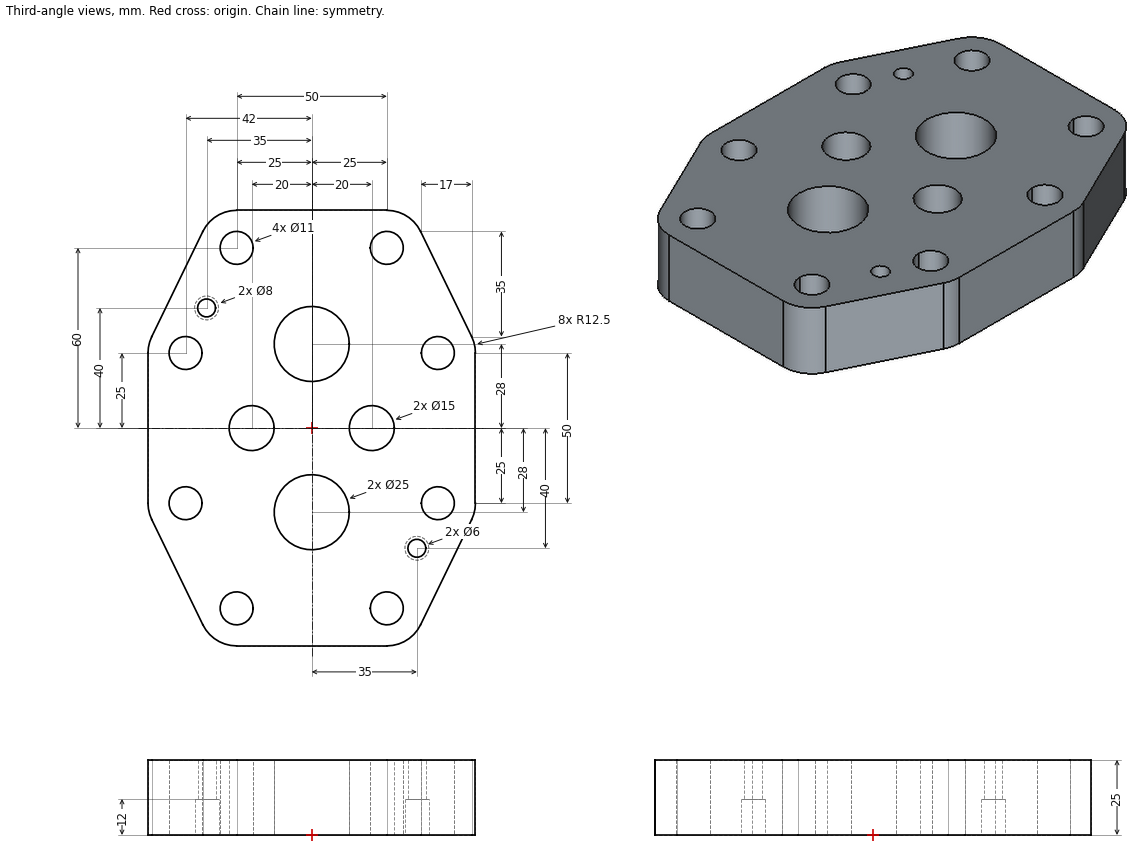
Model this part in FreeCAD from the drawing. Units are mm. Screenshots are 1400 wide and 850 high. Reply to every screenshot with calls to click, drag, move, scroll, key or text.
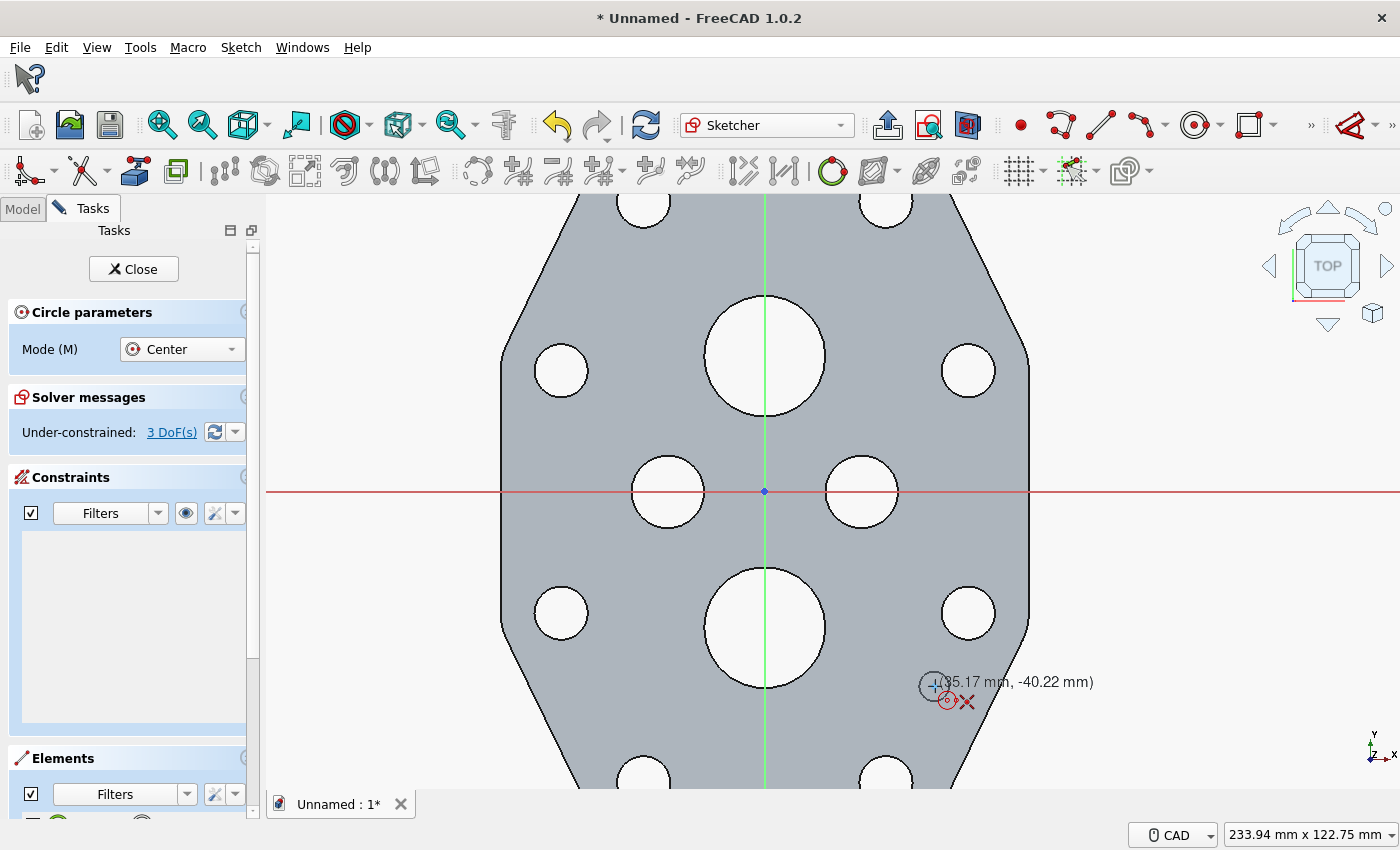
scroll(595, 298, up, 3)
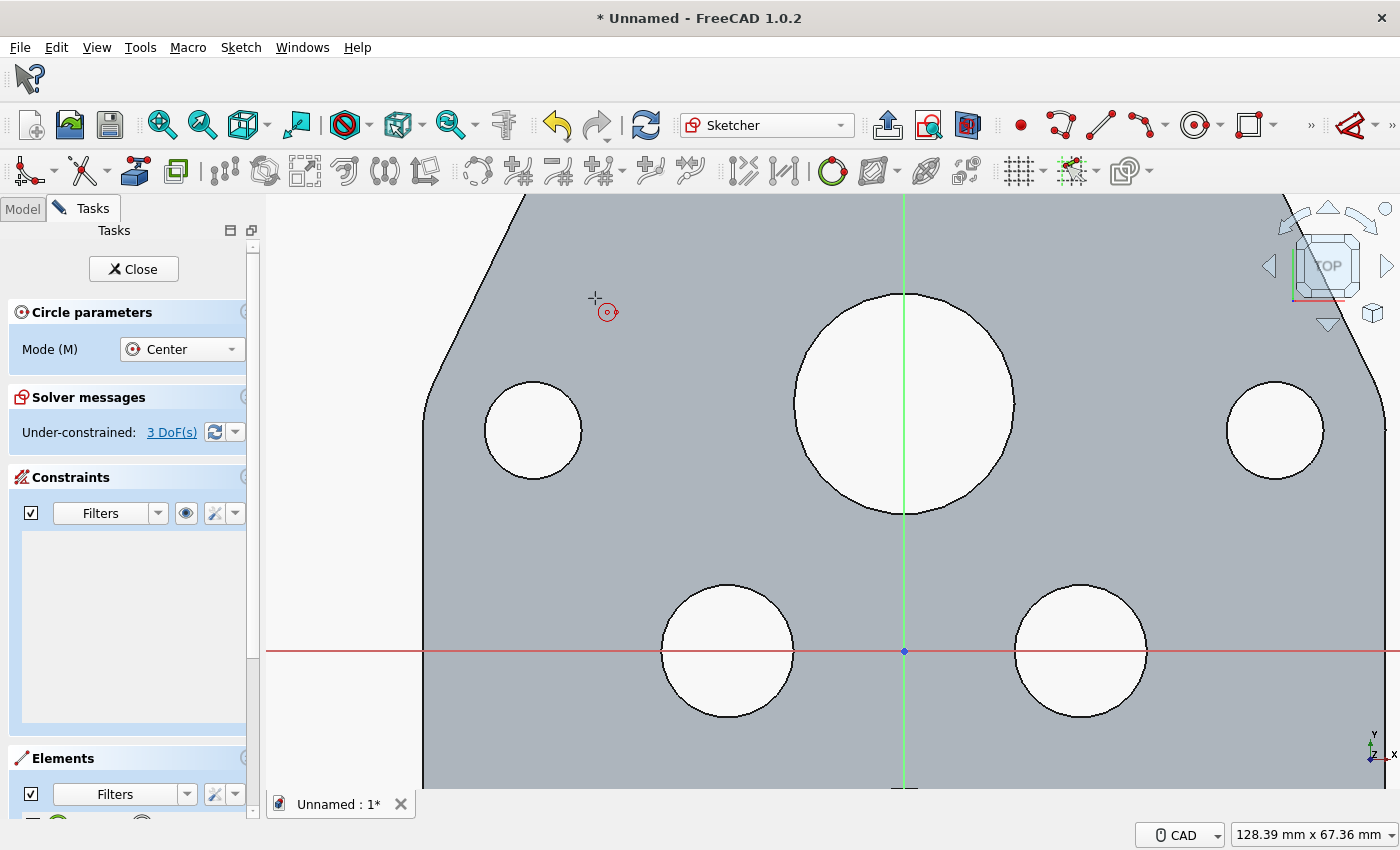
click(595, 298)
click(614, 279)
key(Escape)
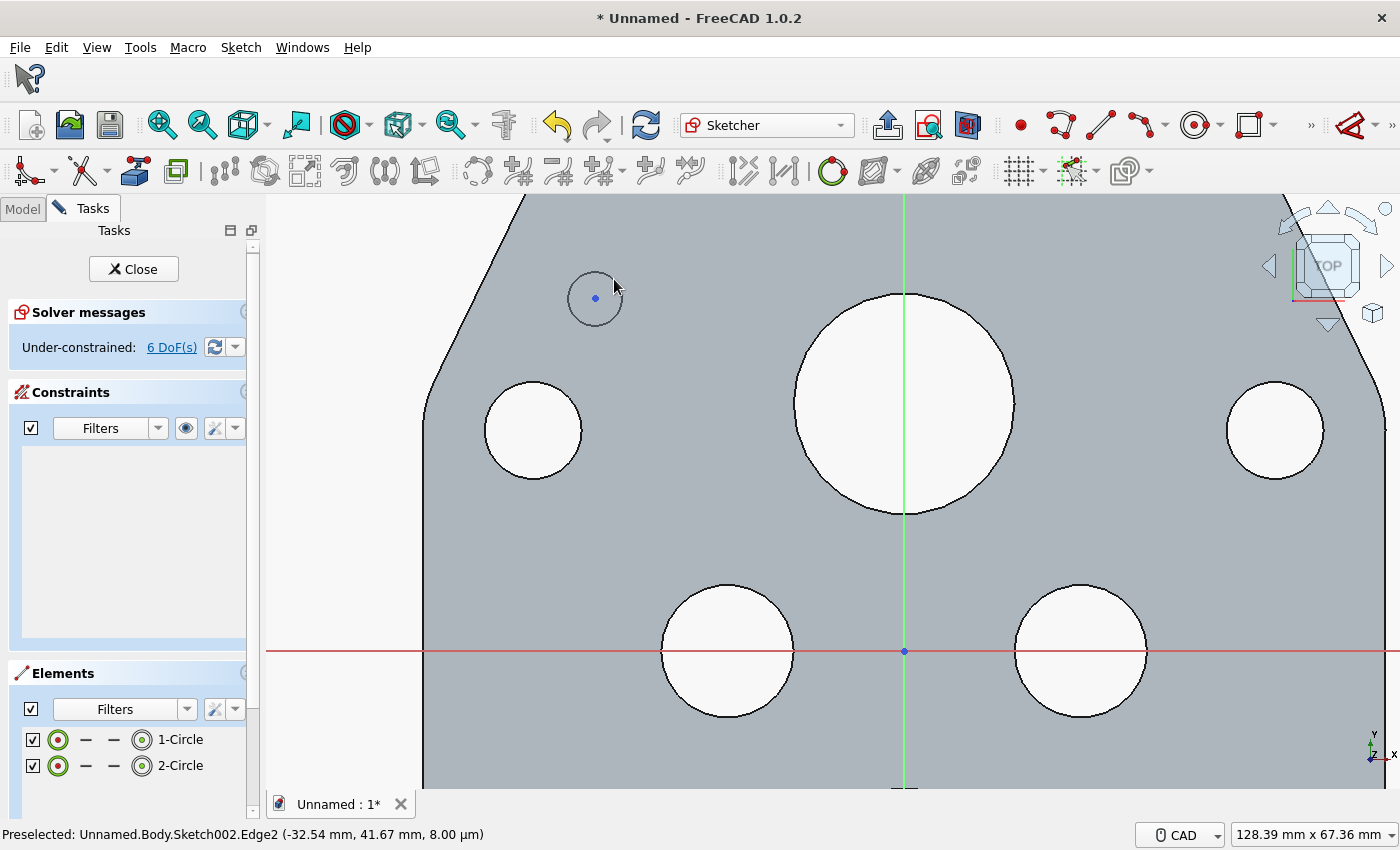
scroll(595, 297, down, 3)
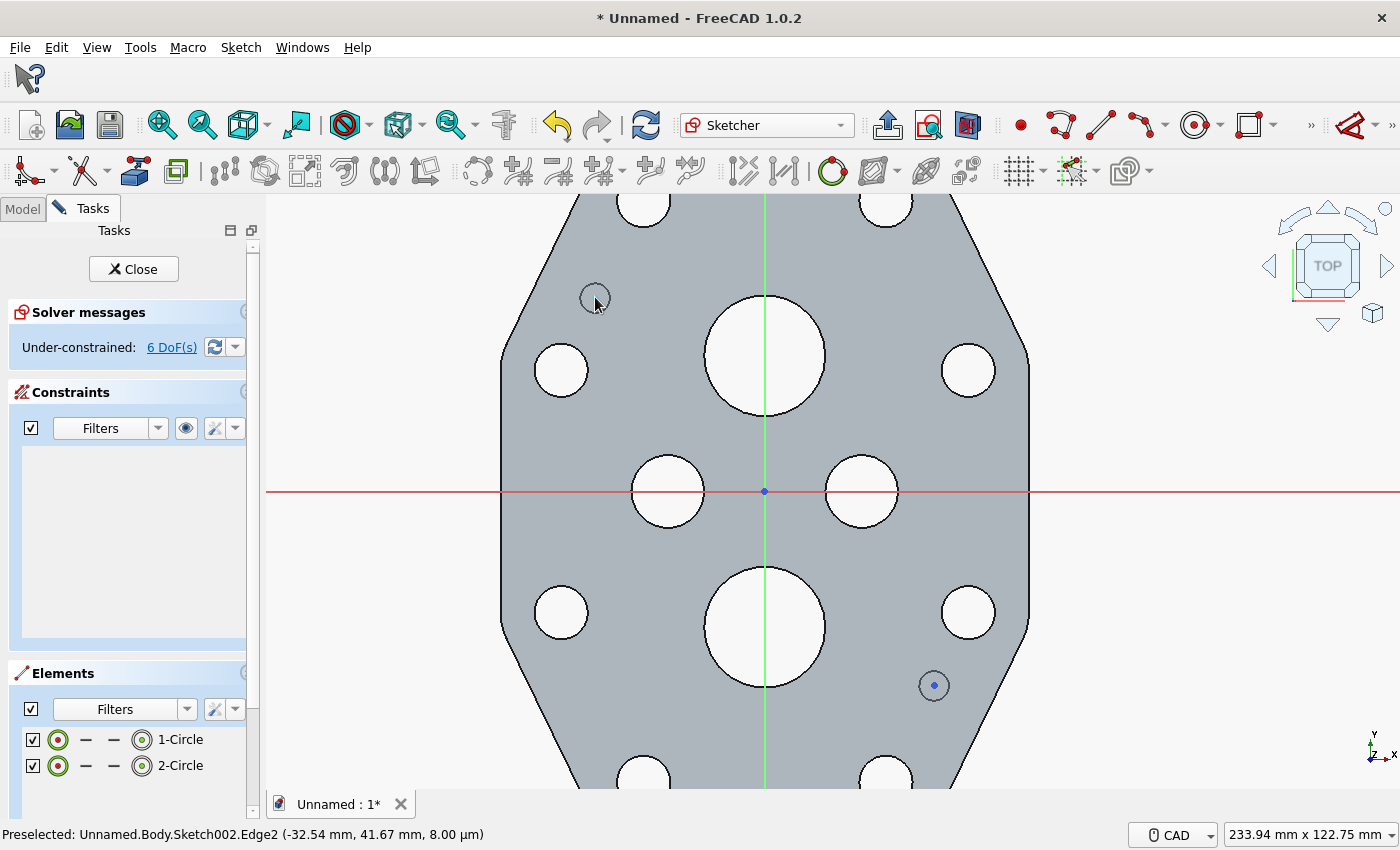
click(945, 675)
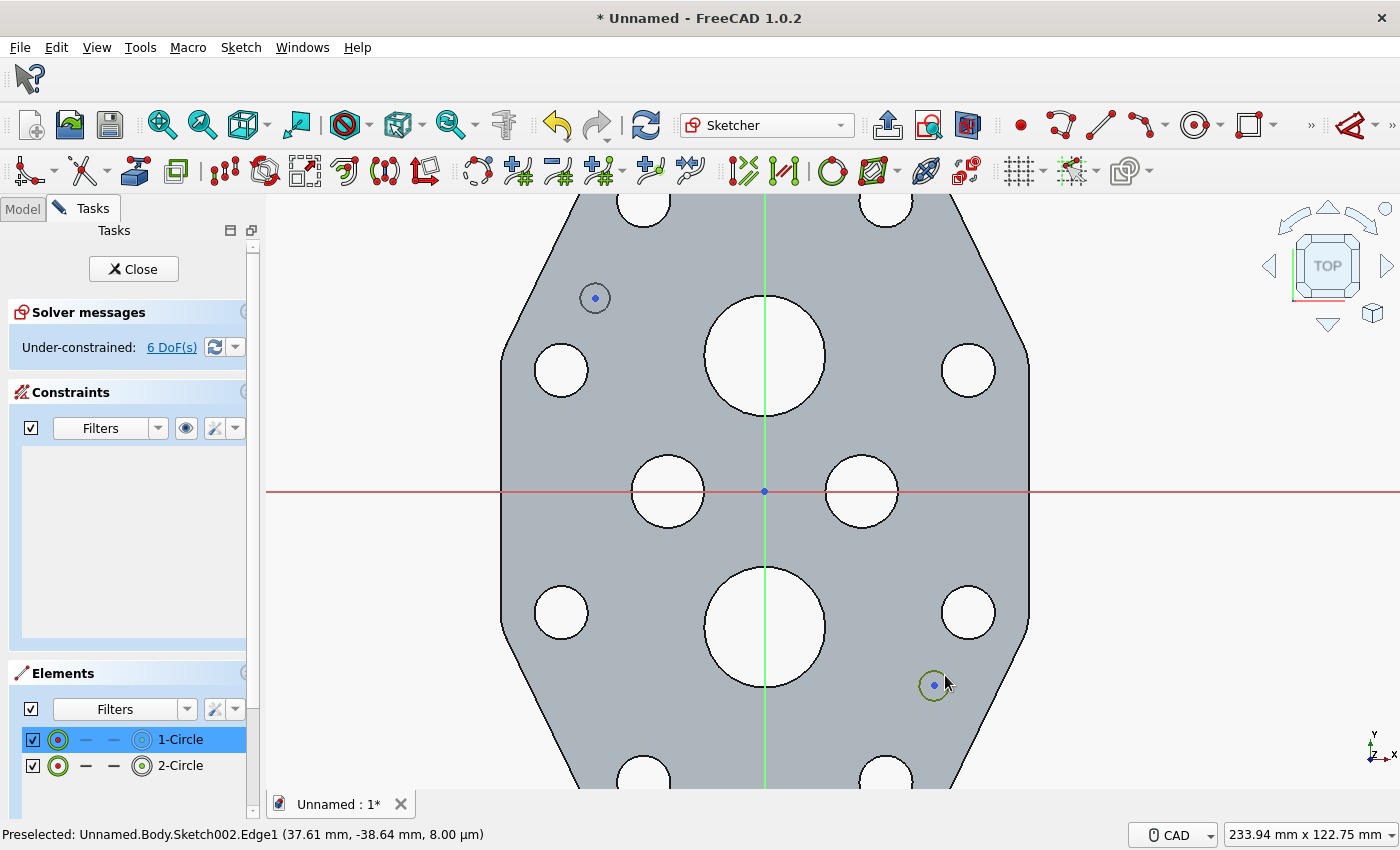
click(606, 288)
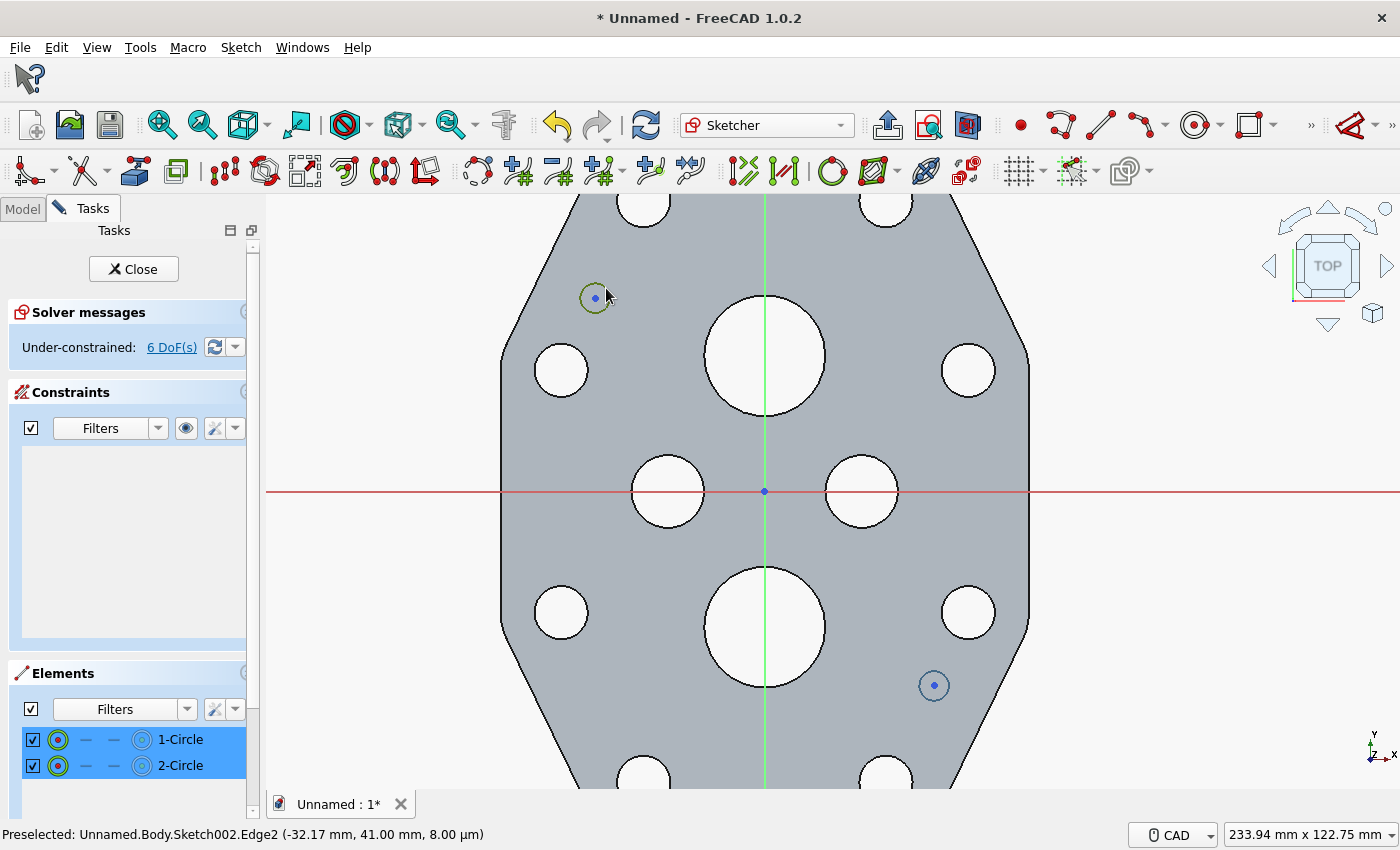
key(e)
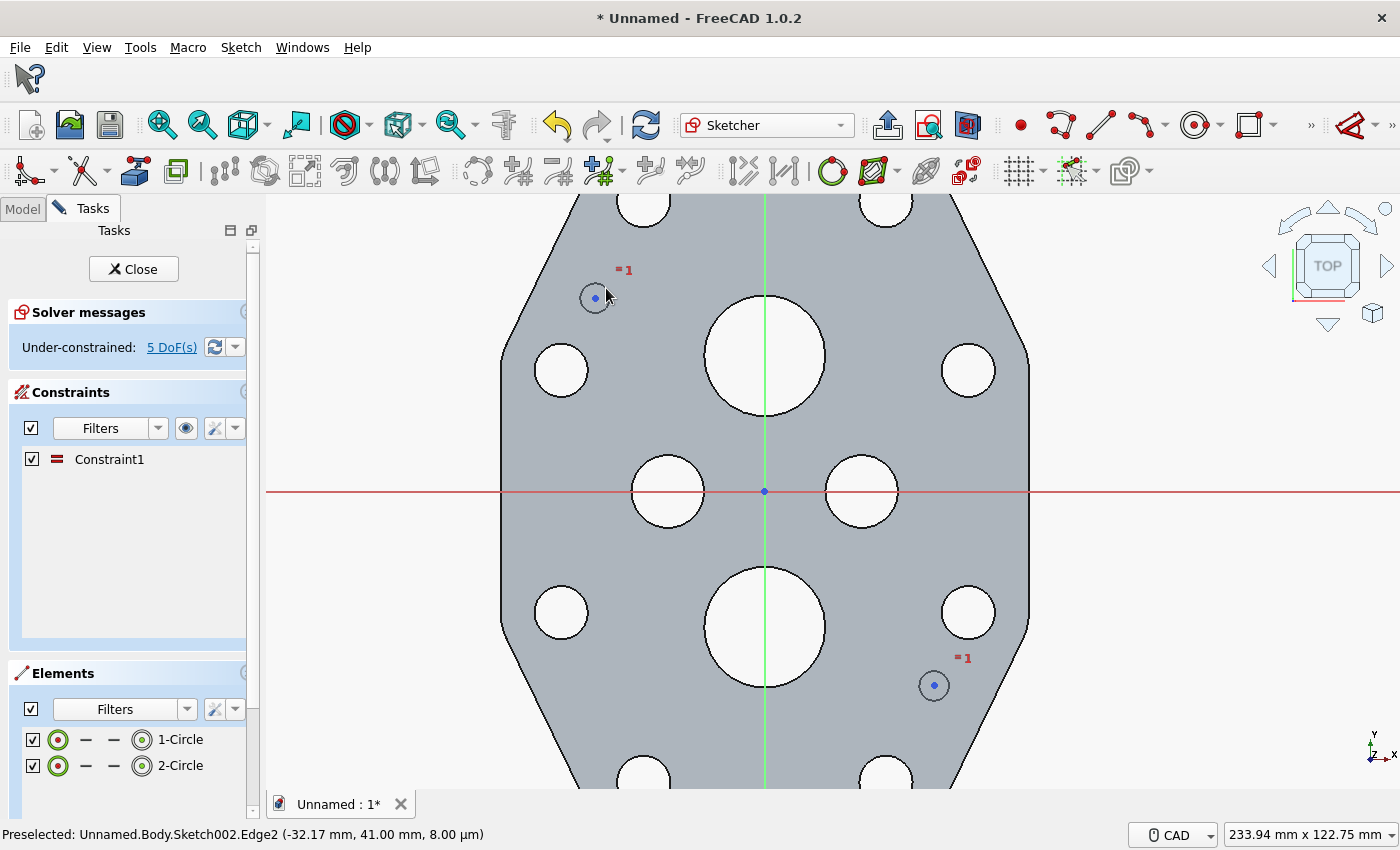
click(1350, 126)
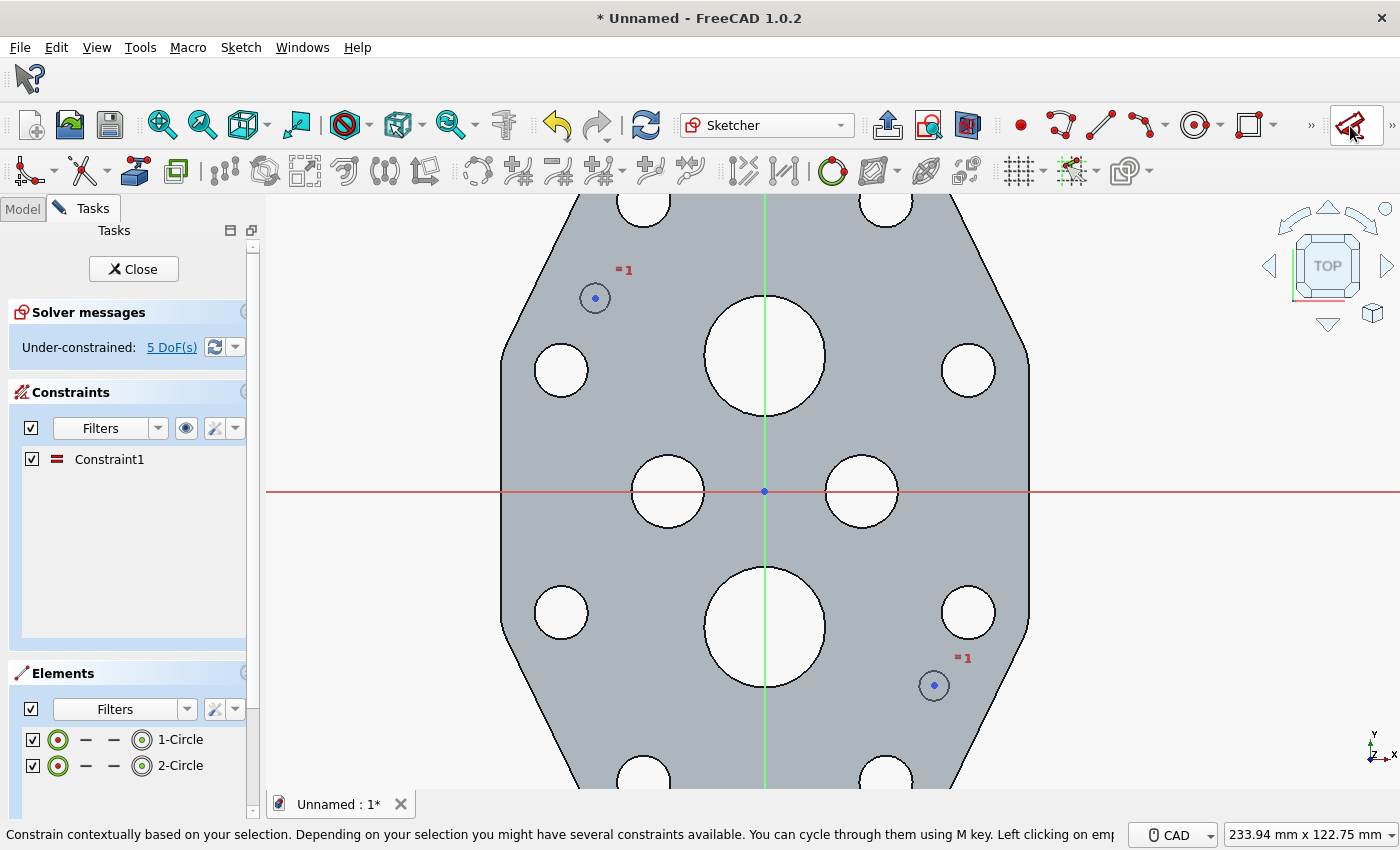
scroll(945, 675, up, 2)